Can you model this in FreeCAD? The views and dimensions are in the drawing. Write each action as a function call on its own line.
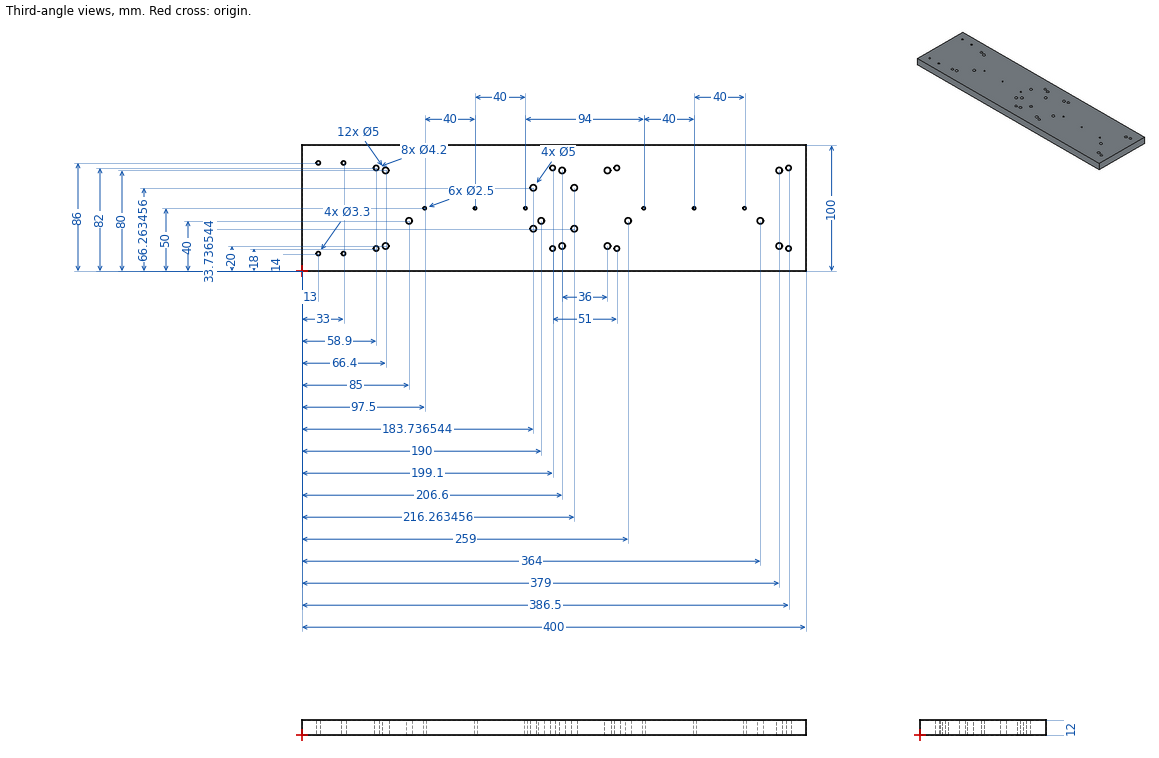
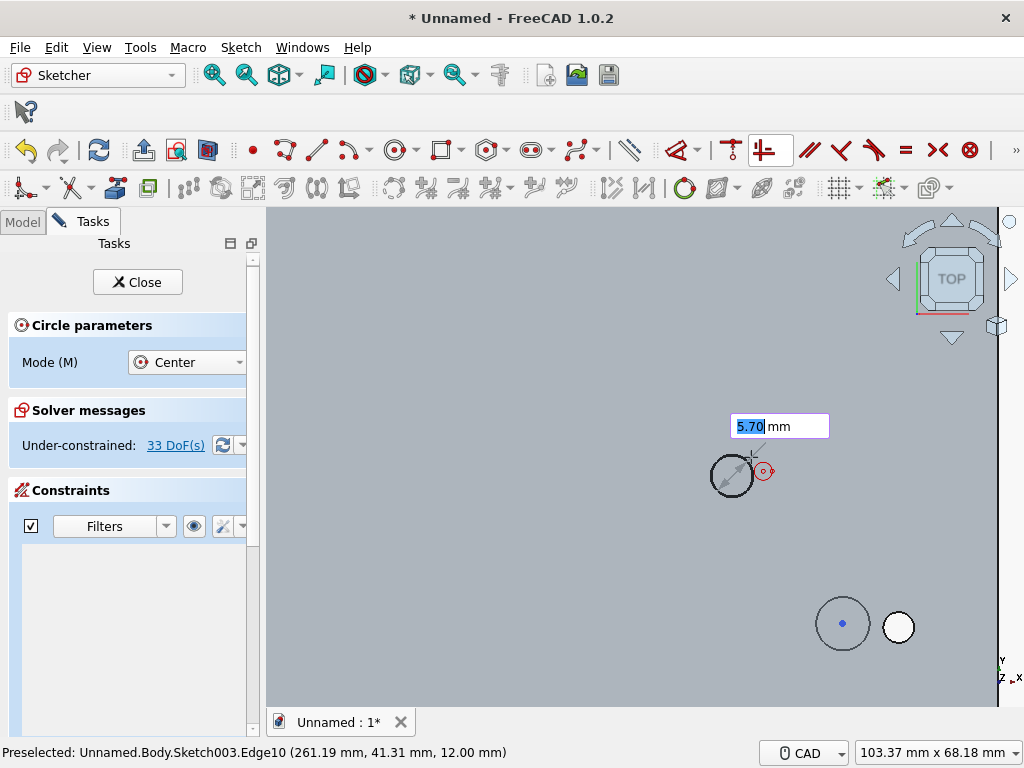
click(747, 453)
key(Escape)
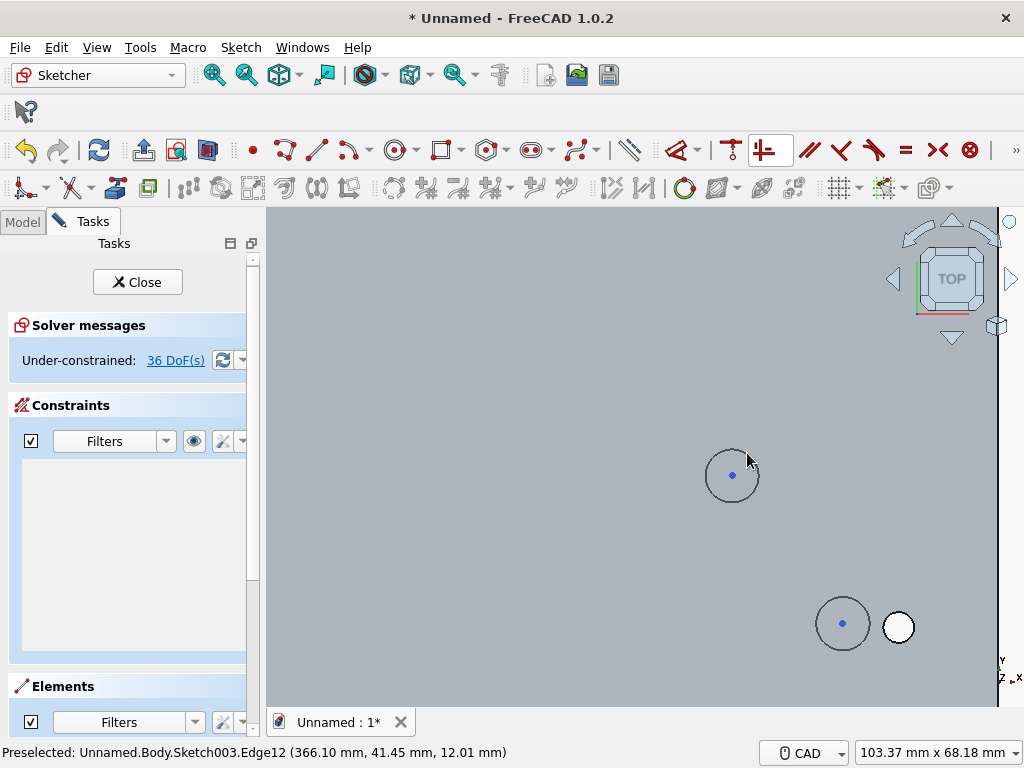
scroll(751, 457, down, 10)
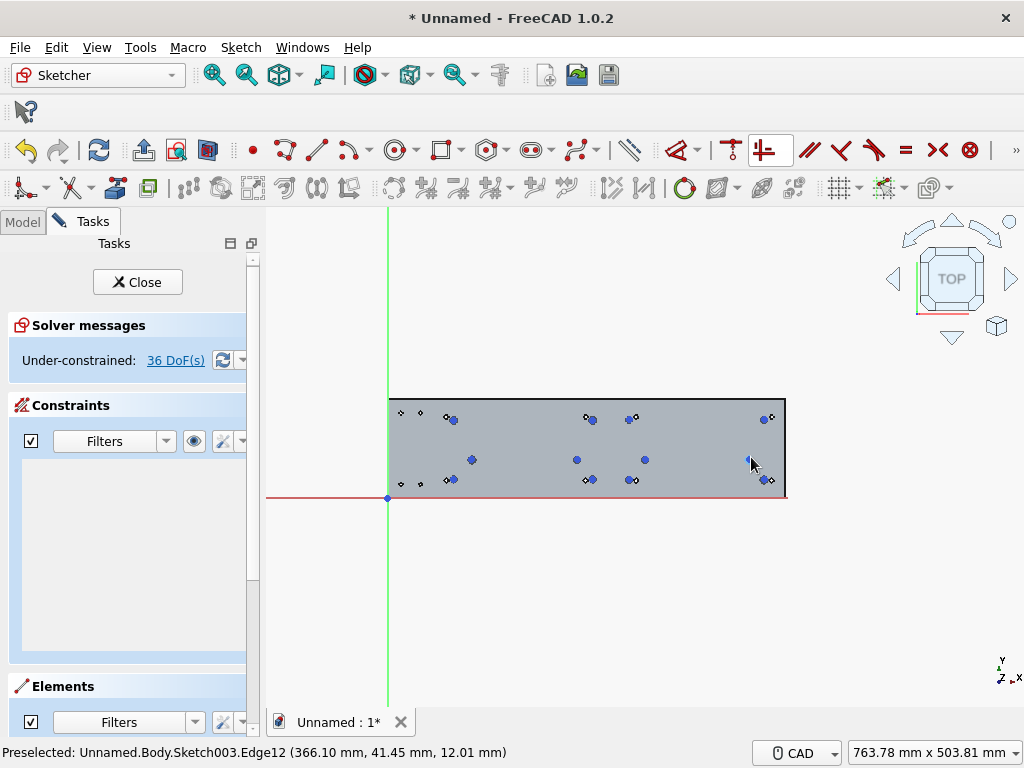
scroll(456, 418, up, 7)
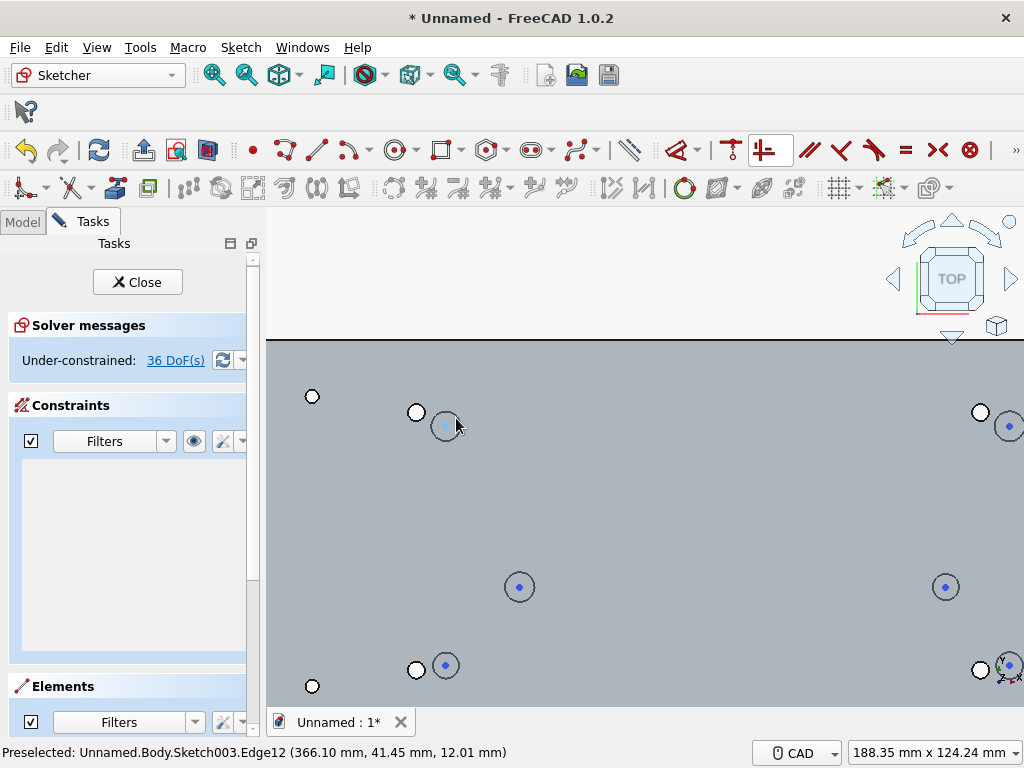
click(456, 416)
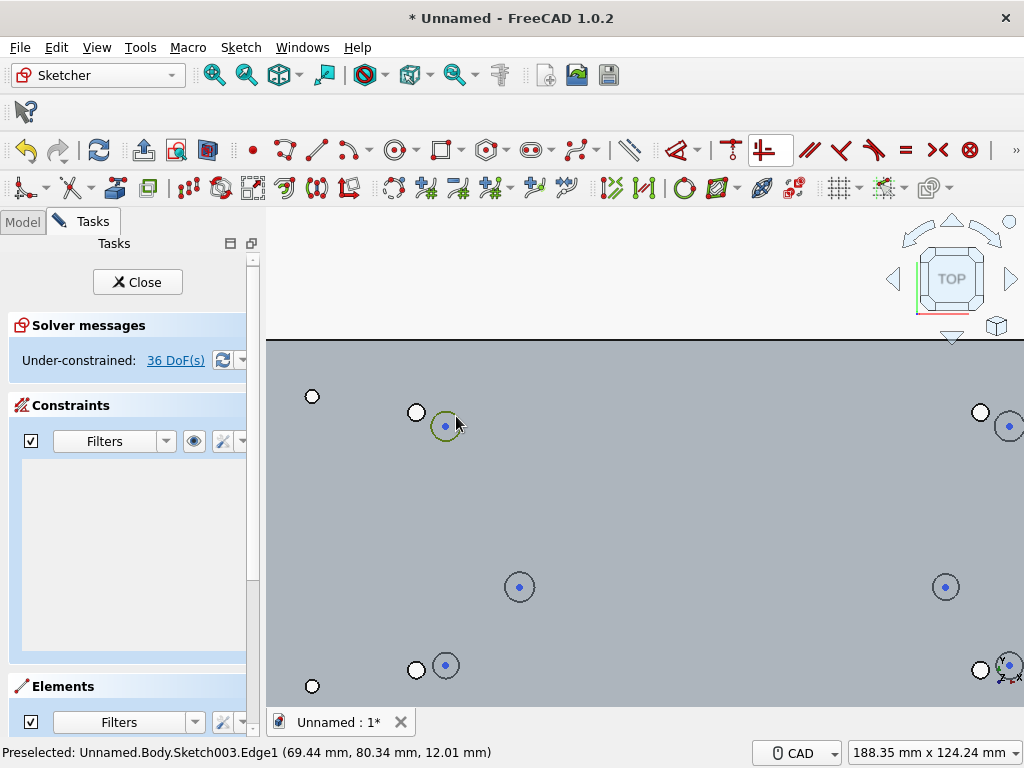
click(455, 656)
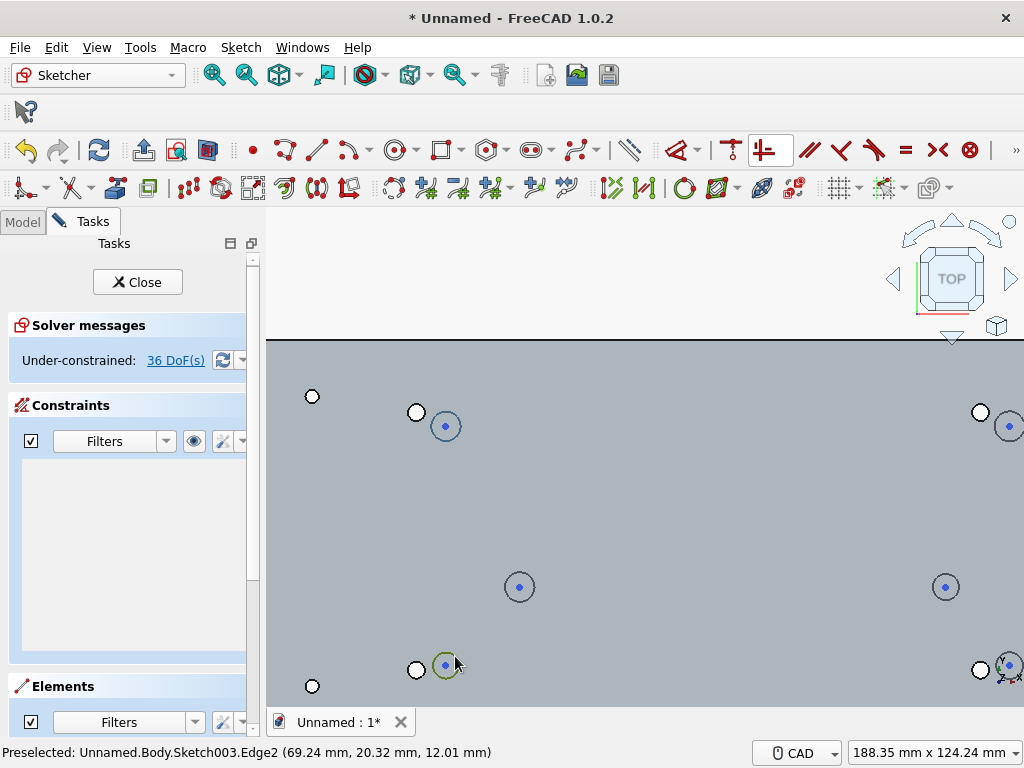
scroll(455, 418, down, 7)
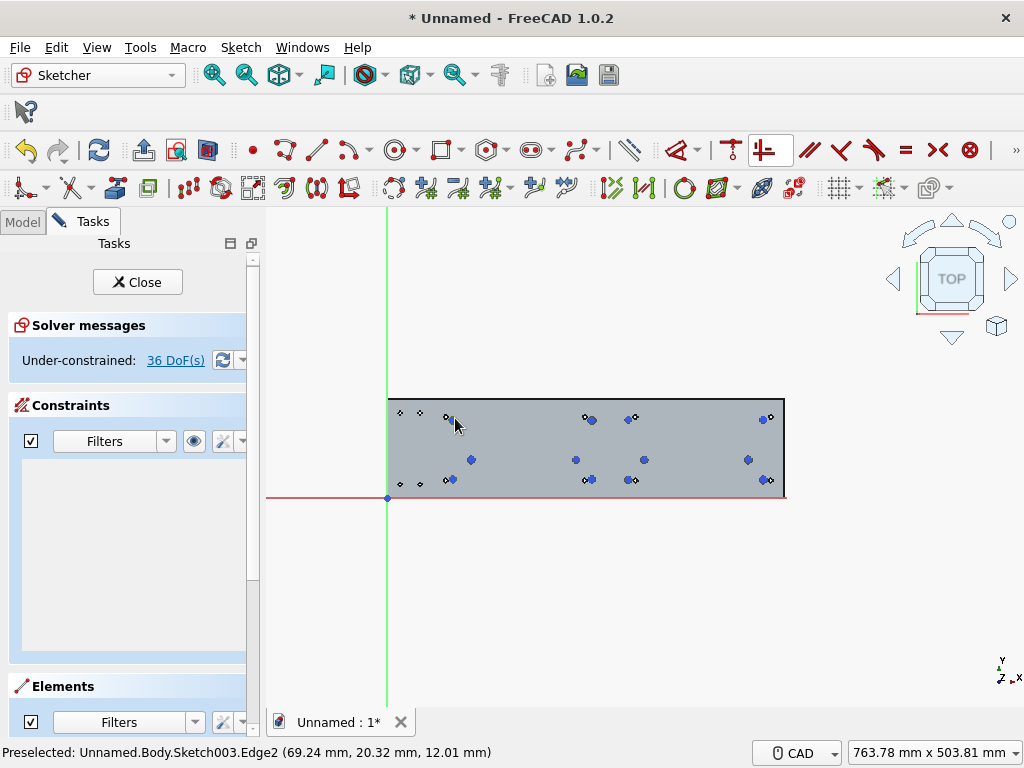
scroll(595, 418, up, 7)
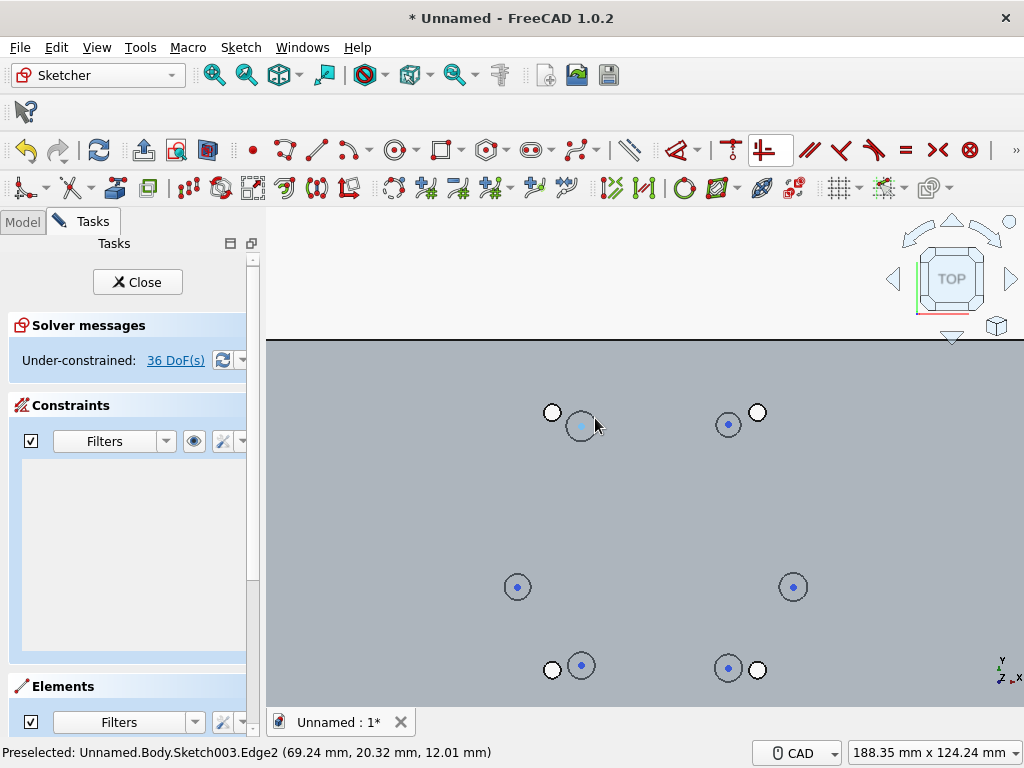
click(592, 416)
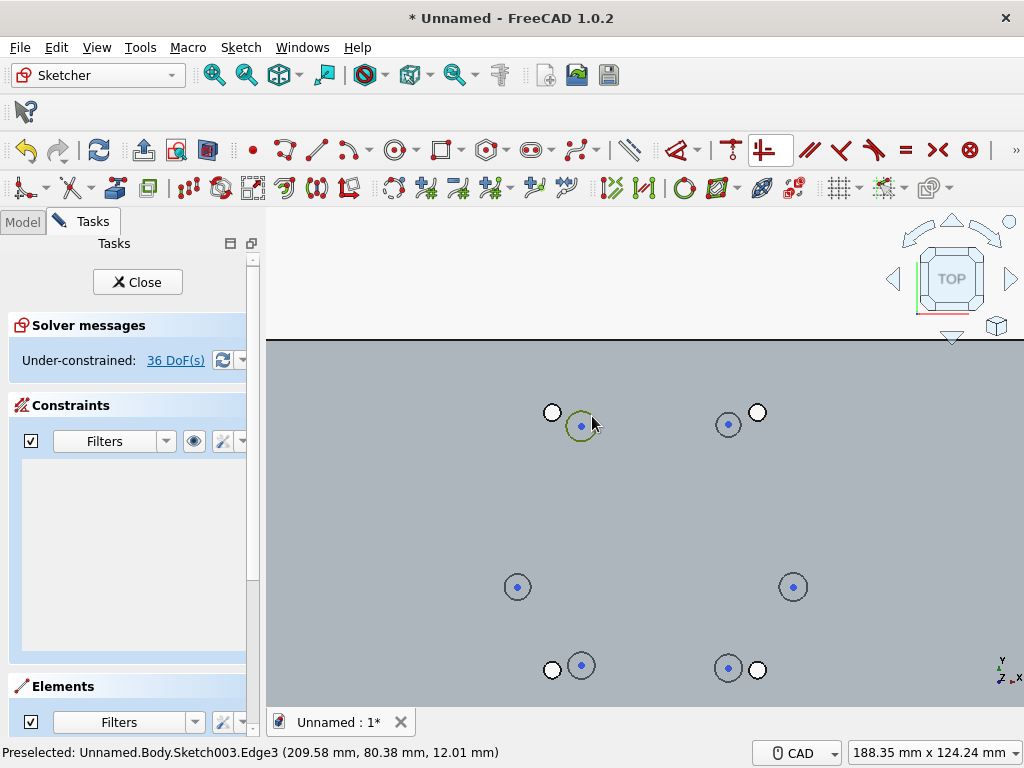
click(591, 656)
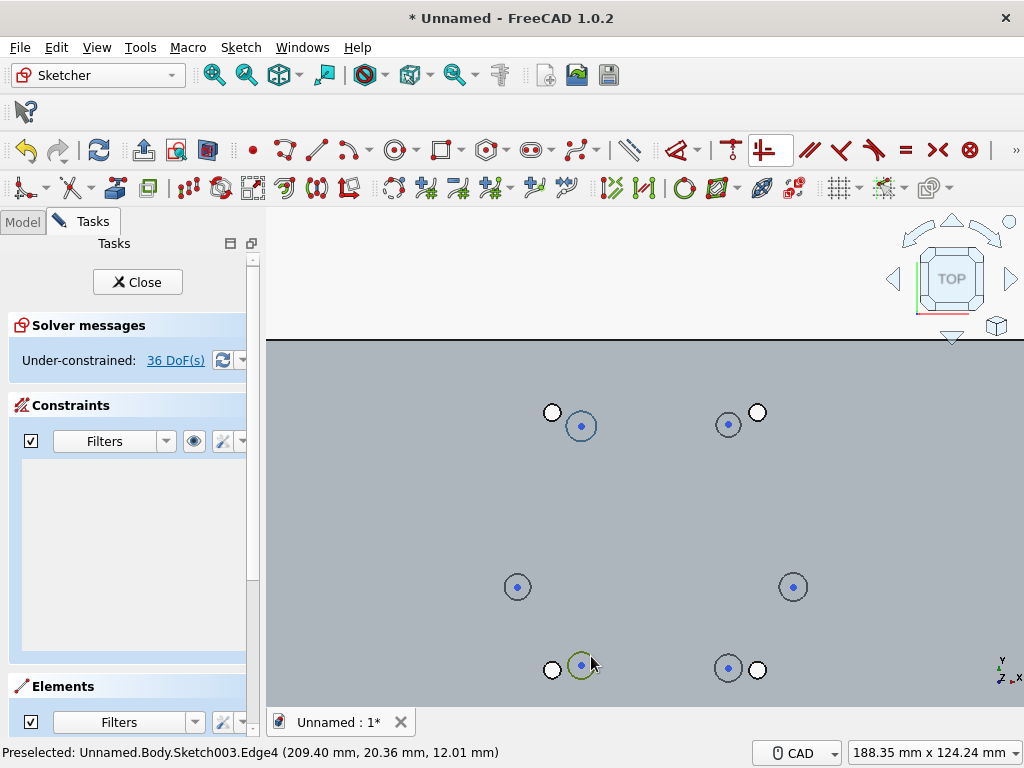
click(738, 658)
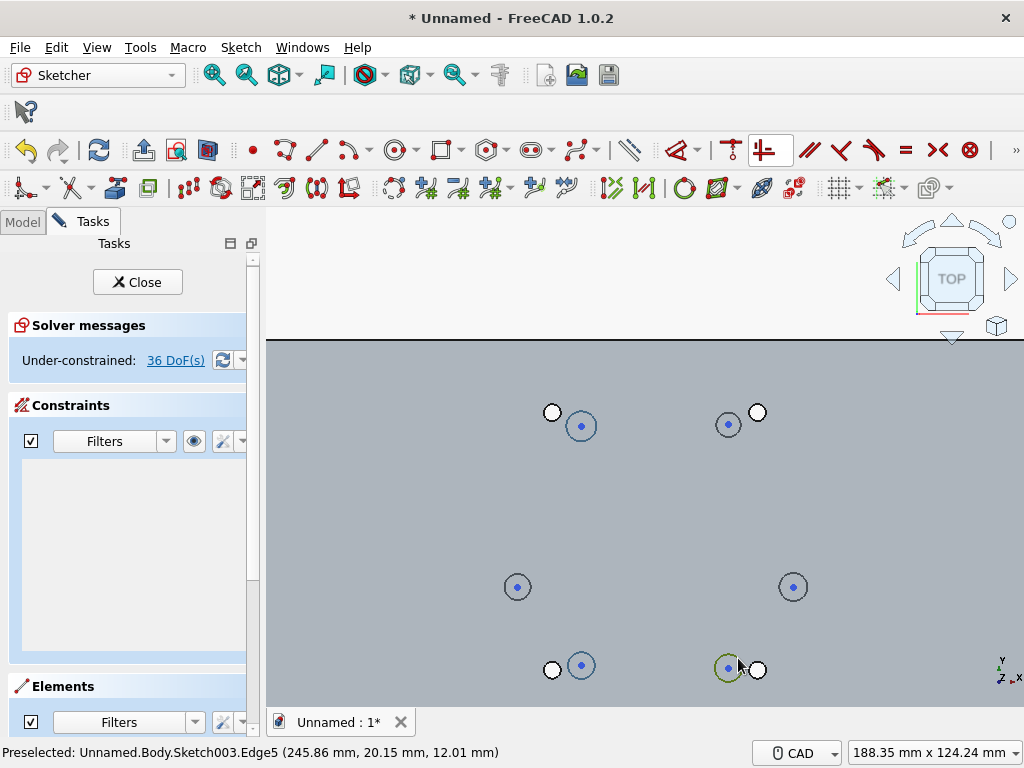
click(737, 416)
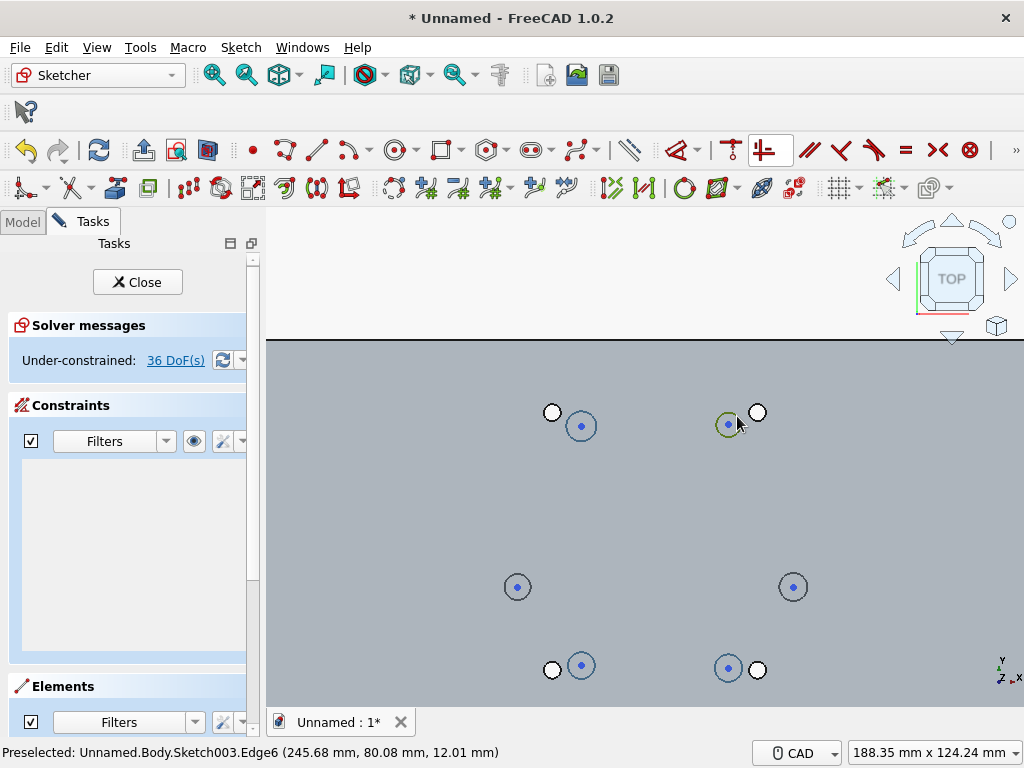
scroll(595, 418, down, 7)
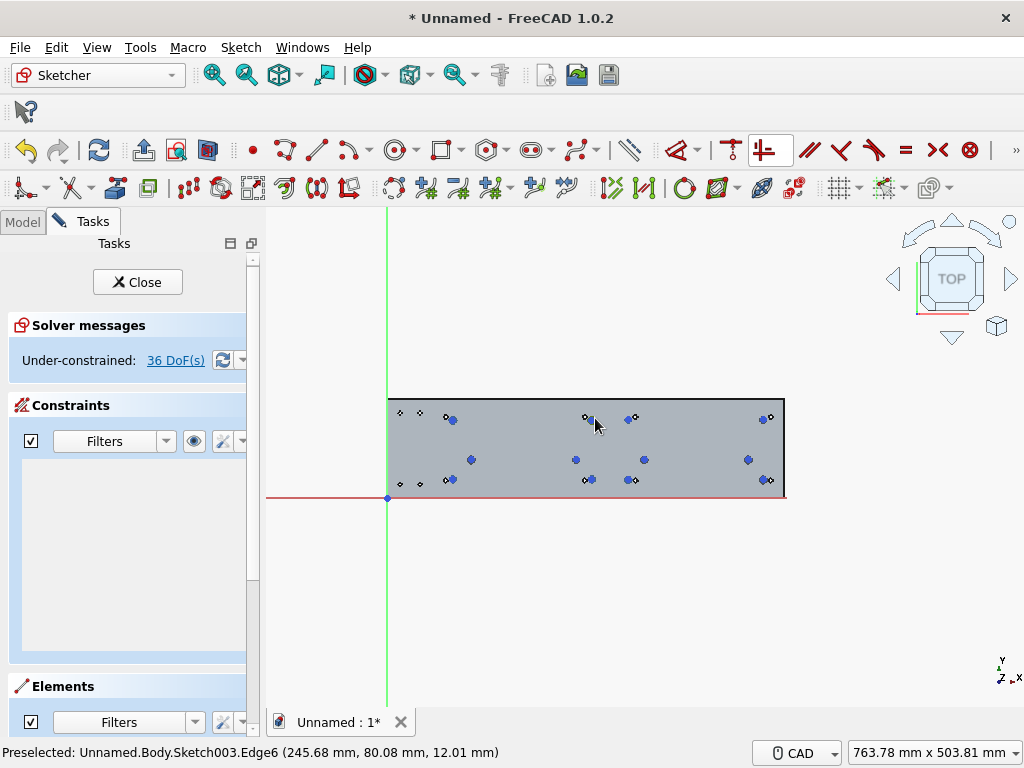
scroll(766, 418, up, 8)